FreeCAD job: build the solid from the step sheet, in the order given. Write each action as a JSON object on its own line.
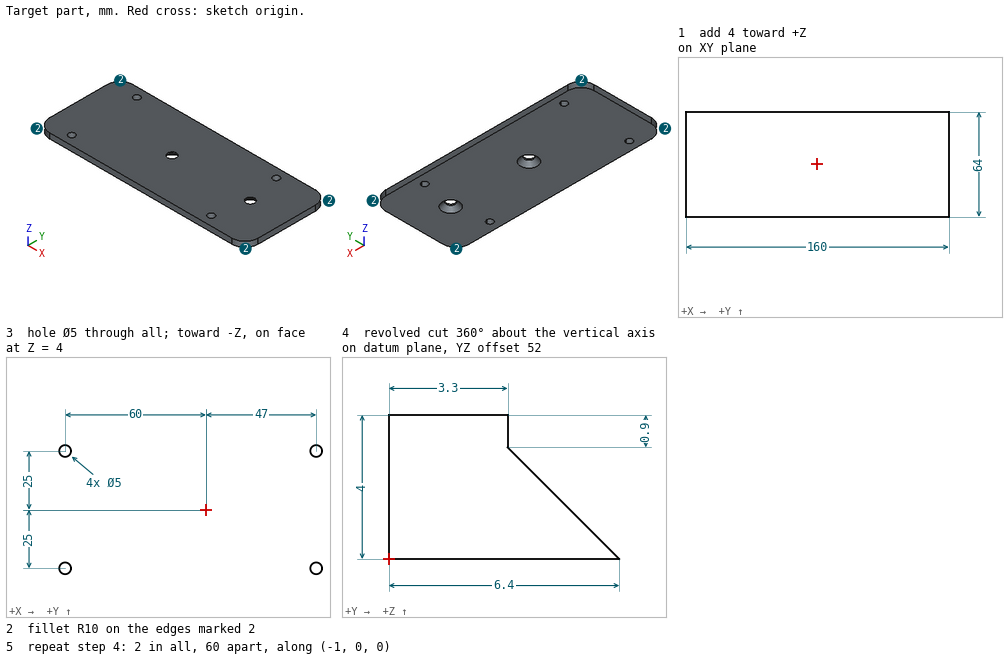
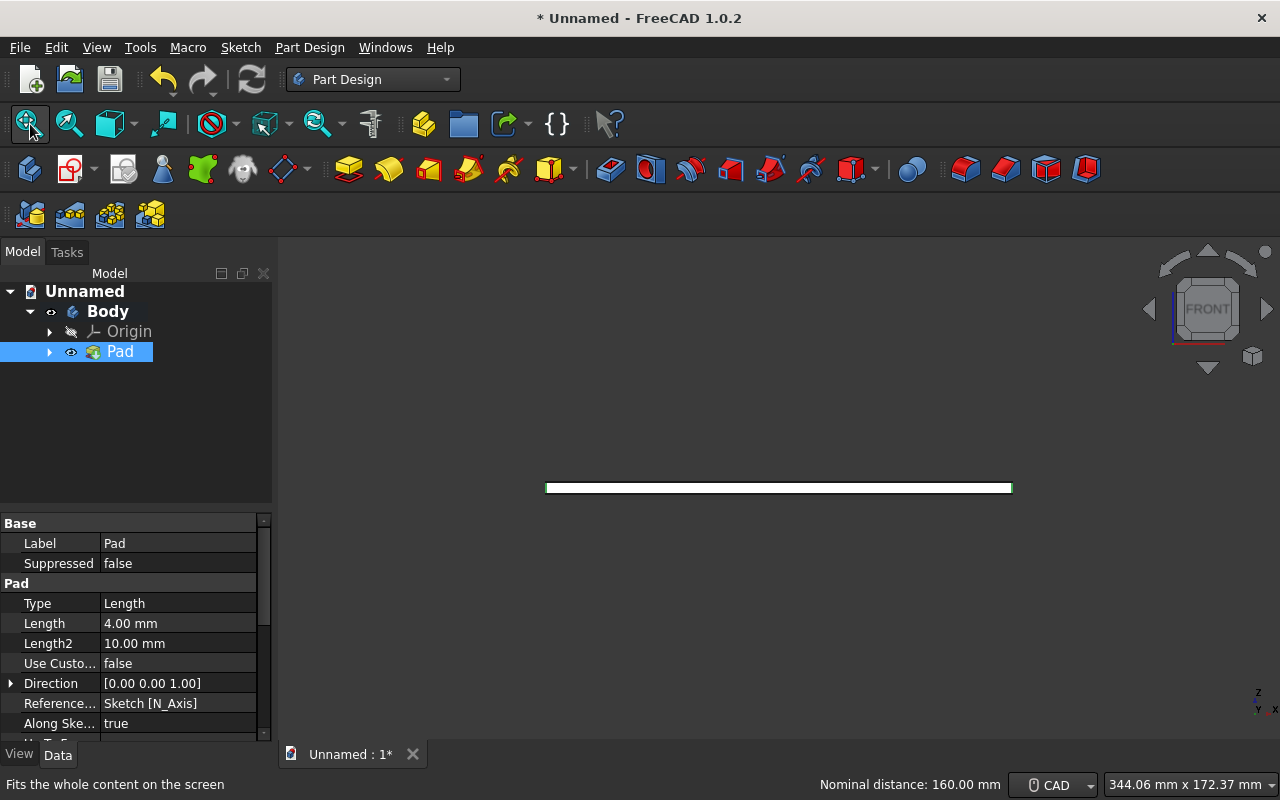
{"action": "key", "text": "3"}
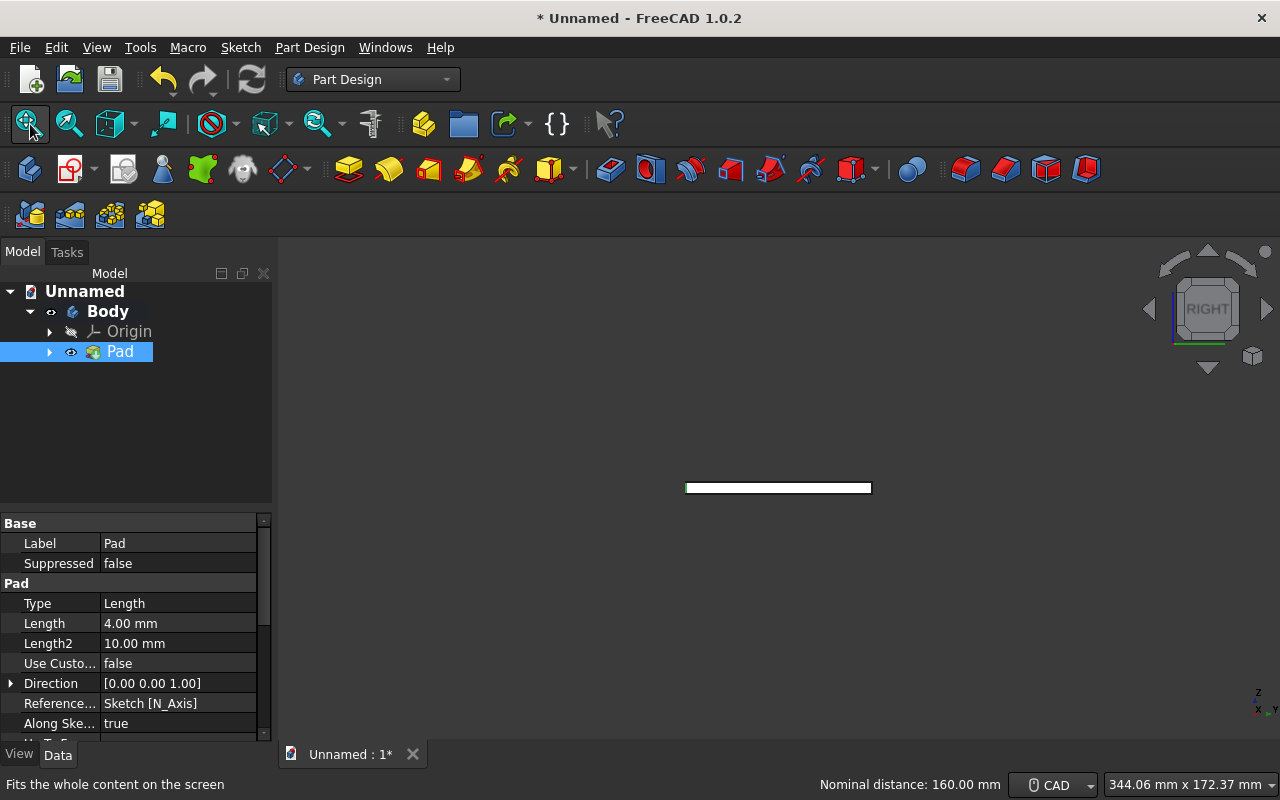
{"action": "left_click", "coordinate": [30, 124]}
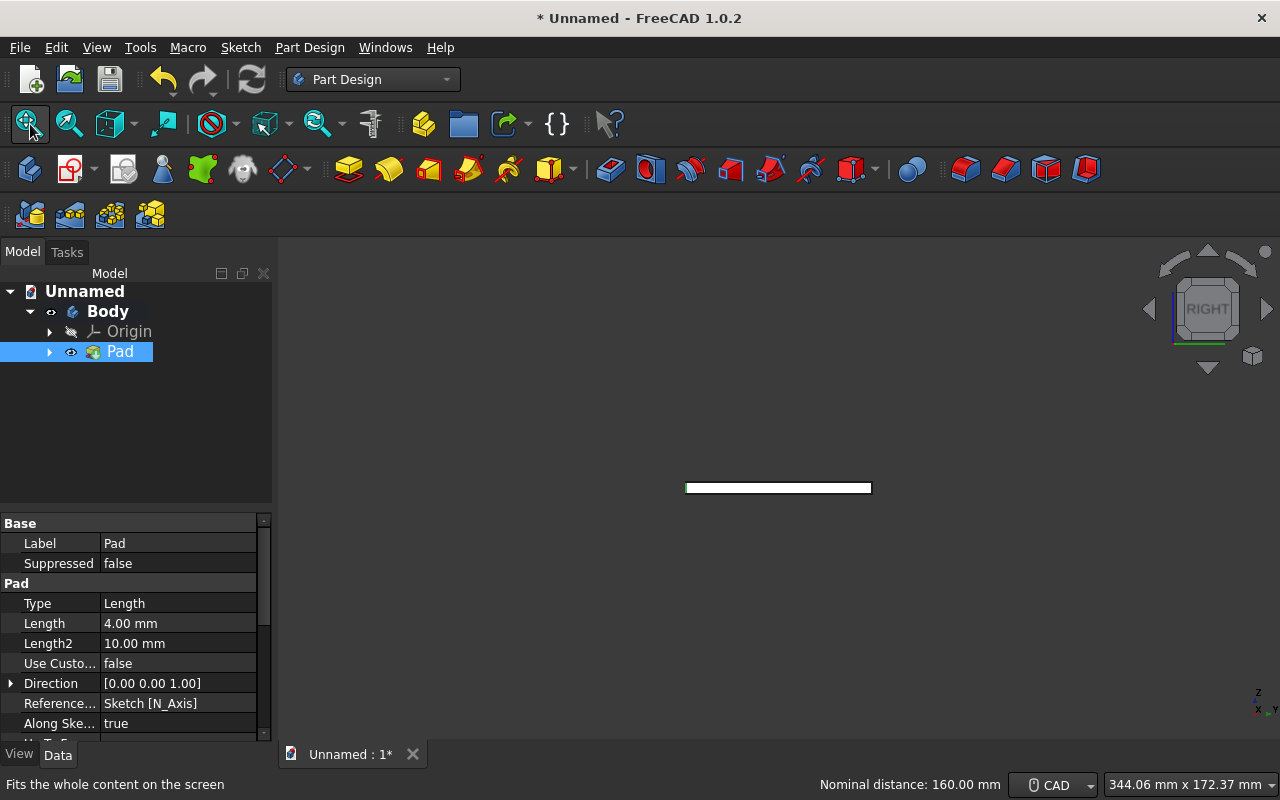
{"action": "scroll", "coordinate": [872, 487], "scroll_direction": "up", "scroll_amount": 7}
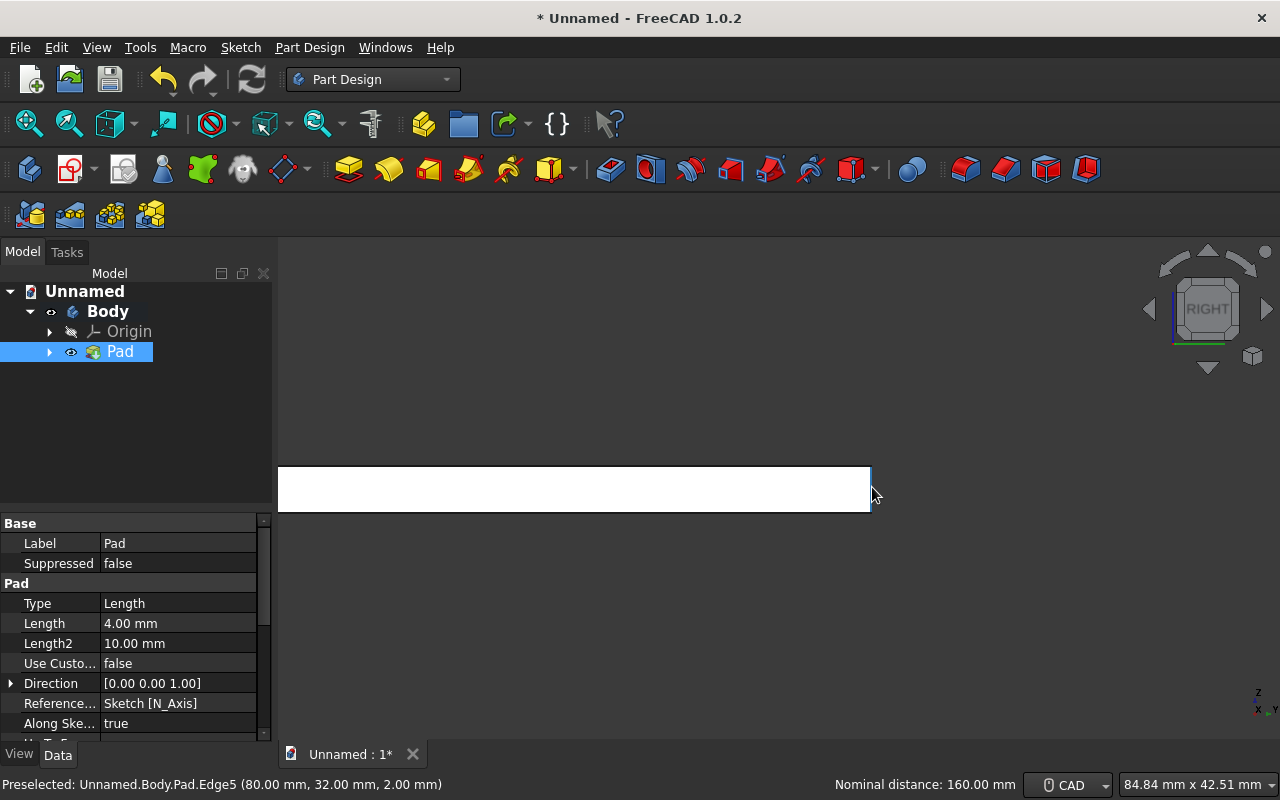
{"action": "left_click", "coordinate": [871, 489], "text": "ctrl"}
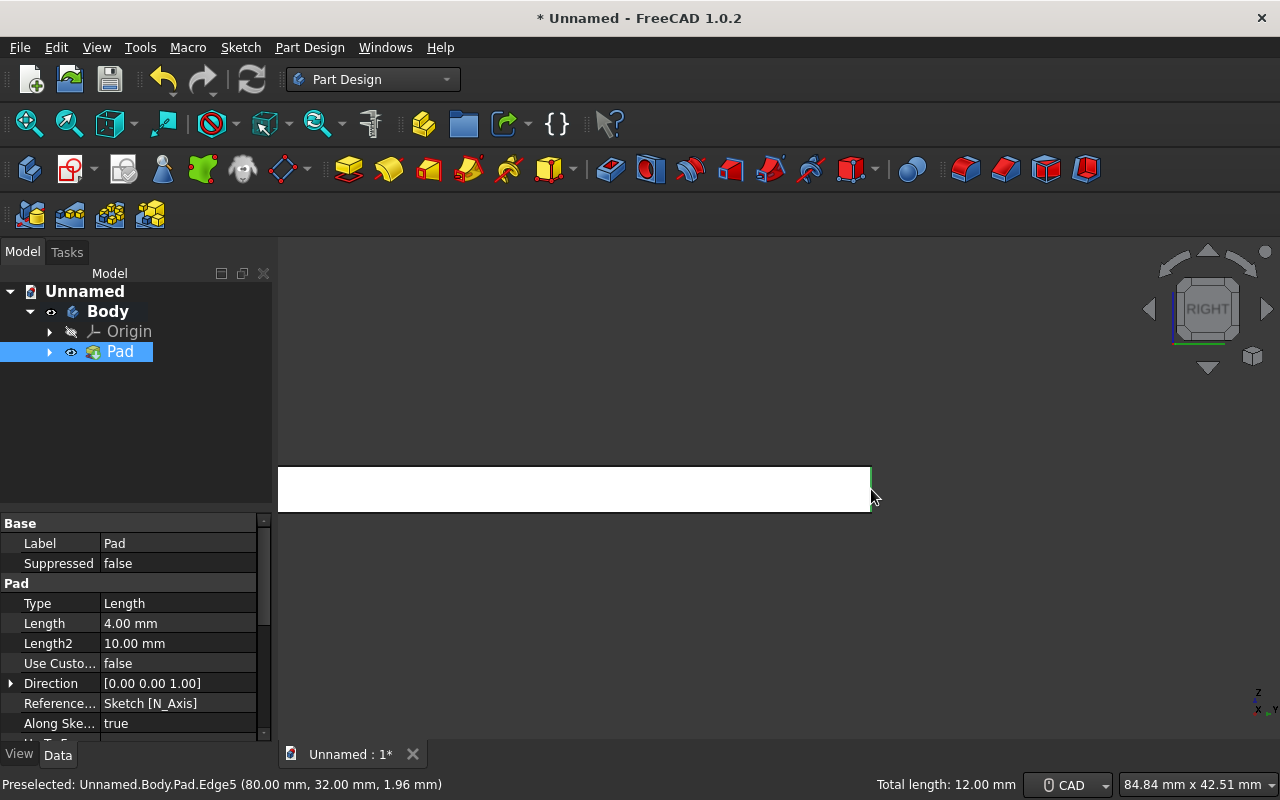
{"action": "left_click", "coordinate": [30, 124]}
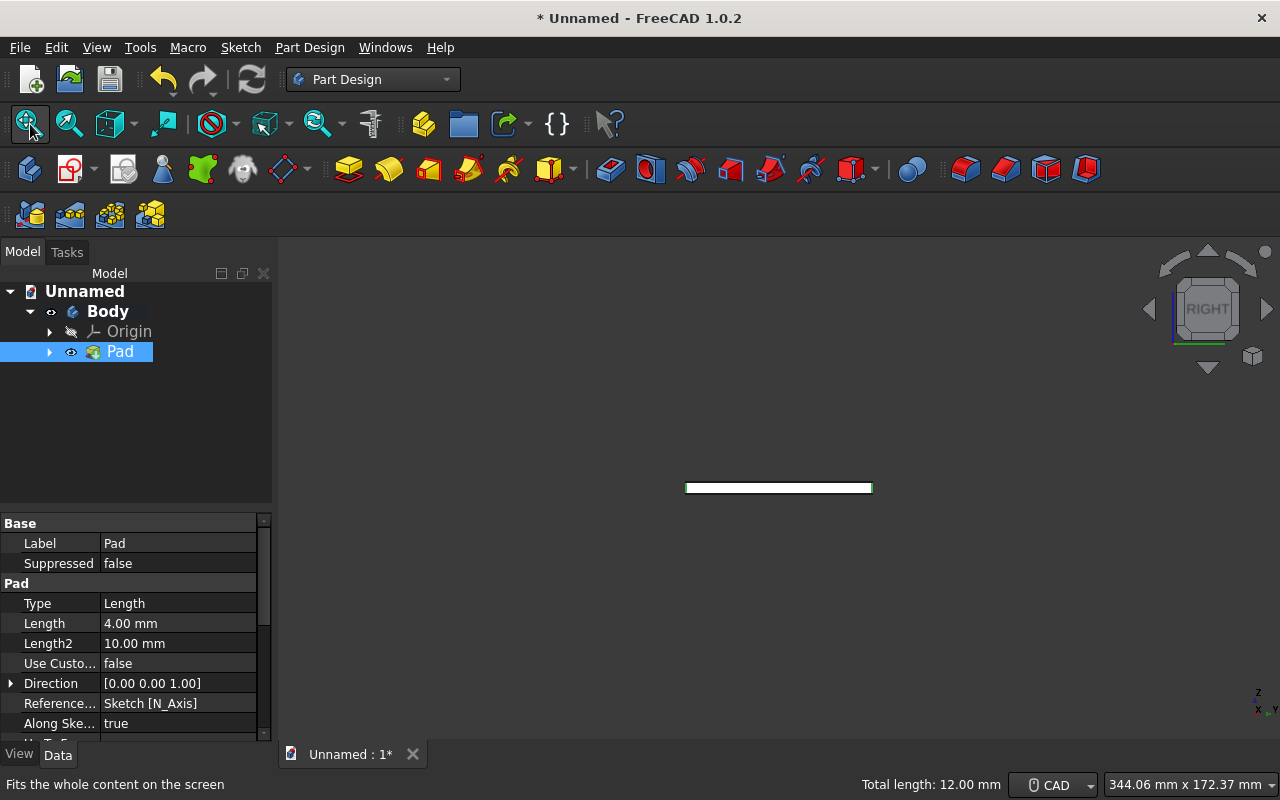
{"action": "key", "text": "5"}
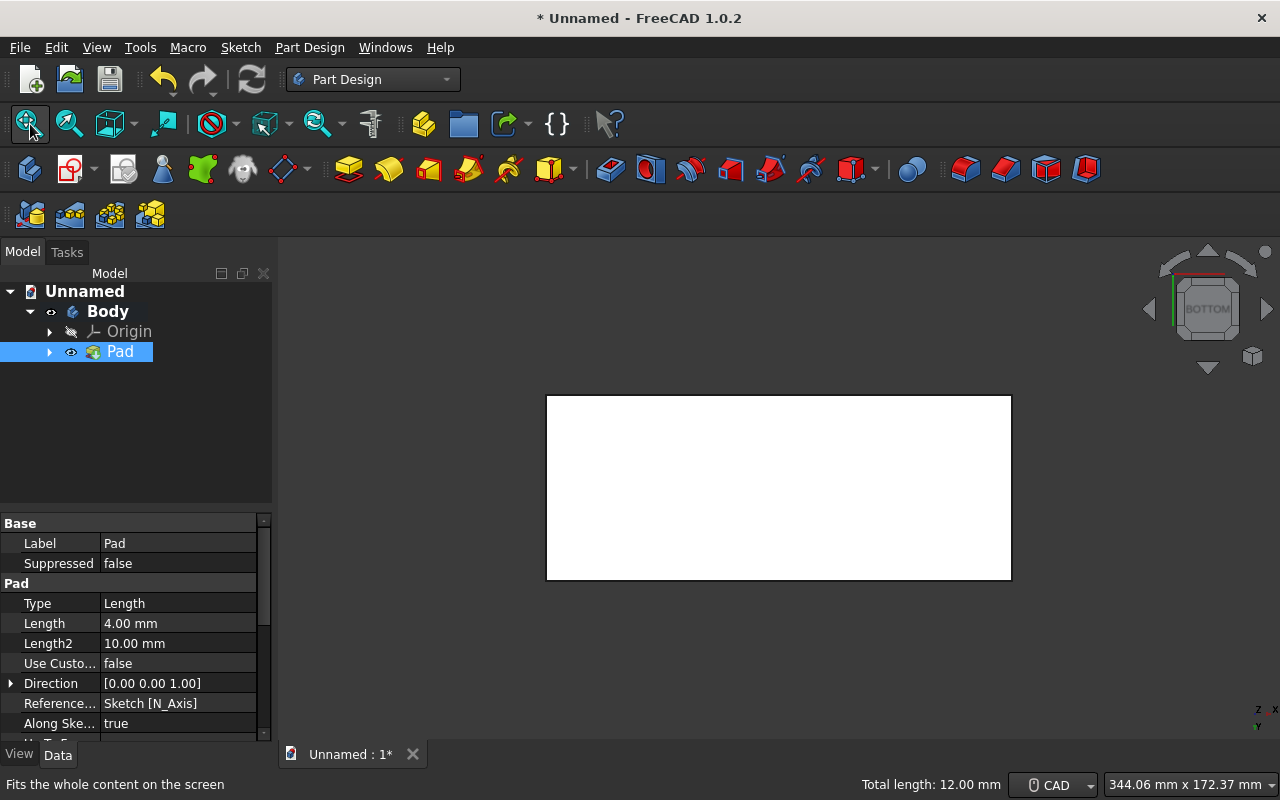
{"action": "scroll", "coordinate": [546, 580], "scroll_direction": "up", "scroll_amount": 7}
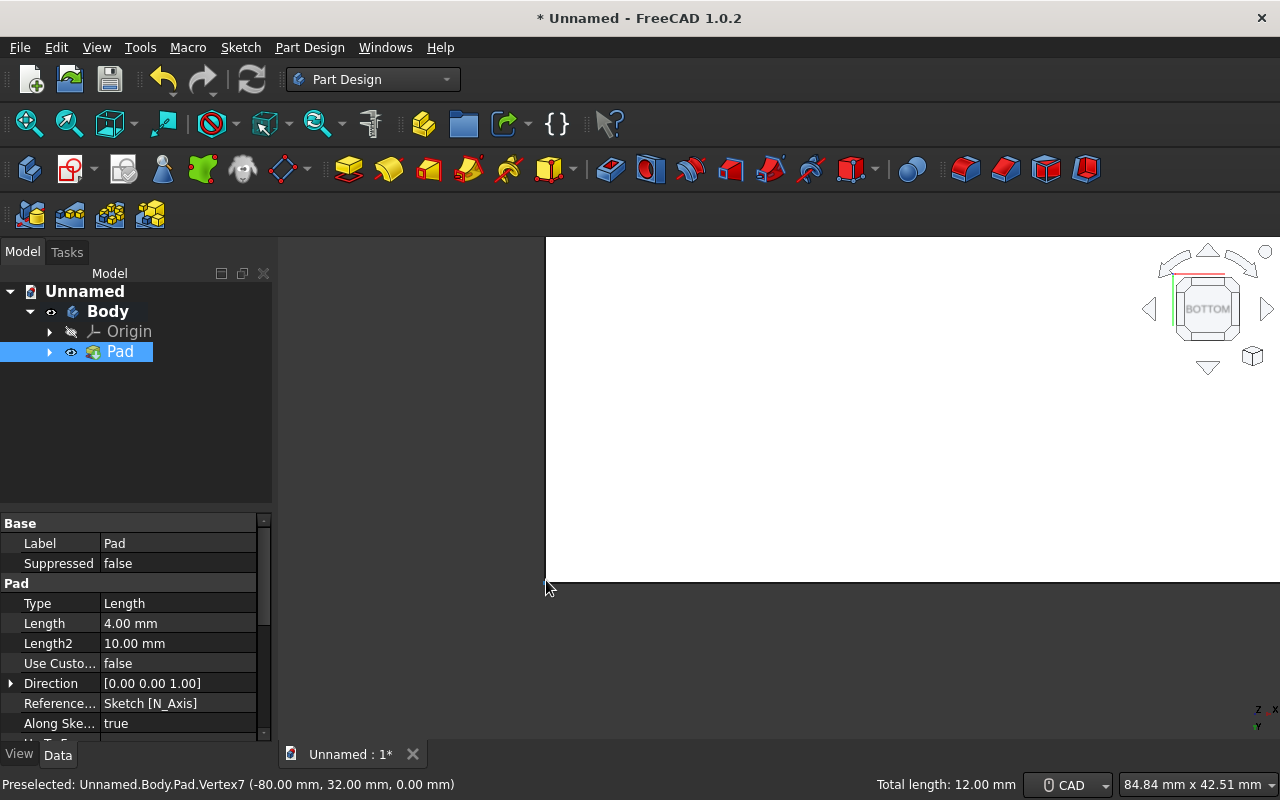
{"action": "left_click", "coordinate": [30, 124]}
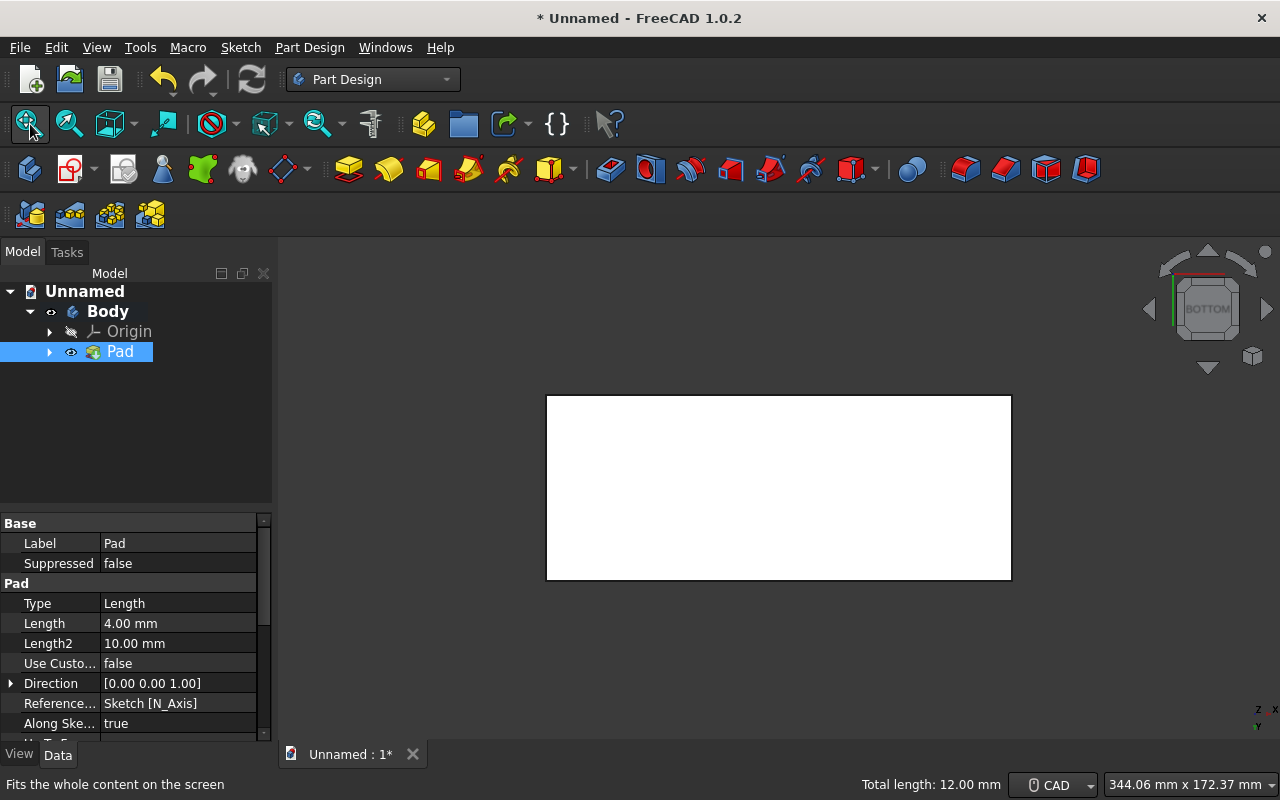
{"action": "key", "text": "4"}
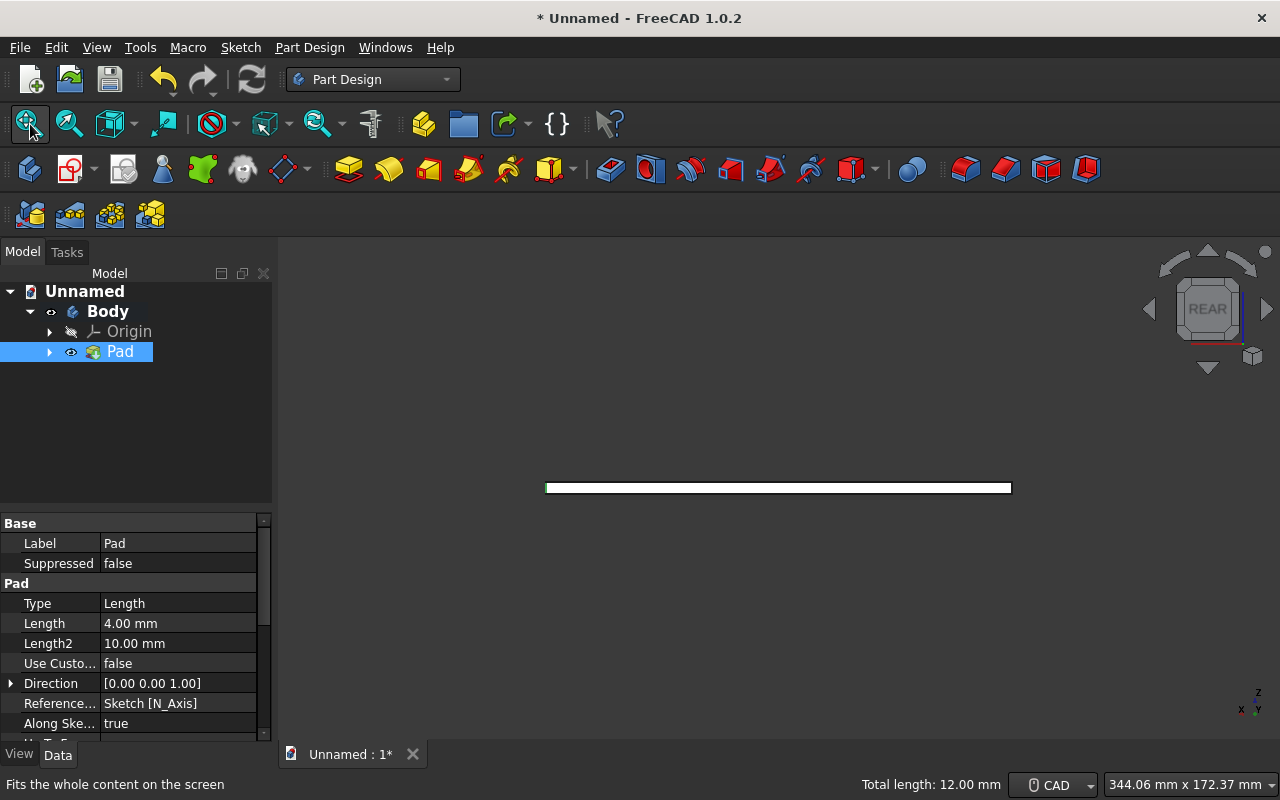
{"action": "scroll", "coordinate": [1012, 487], "scroll_direction": "up", "scroll_amount": 7}